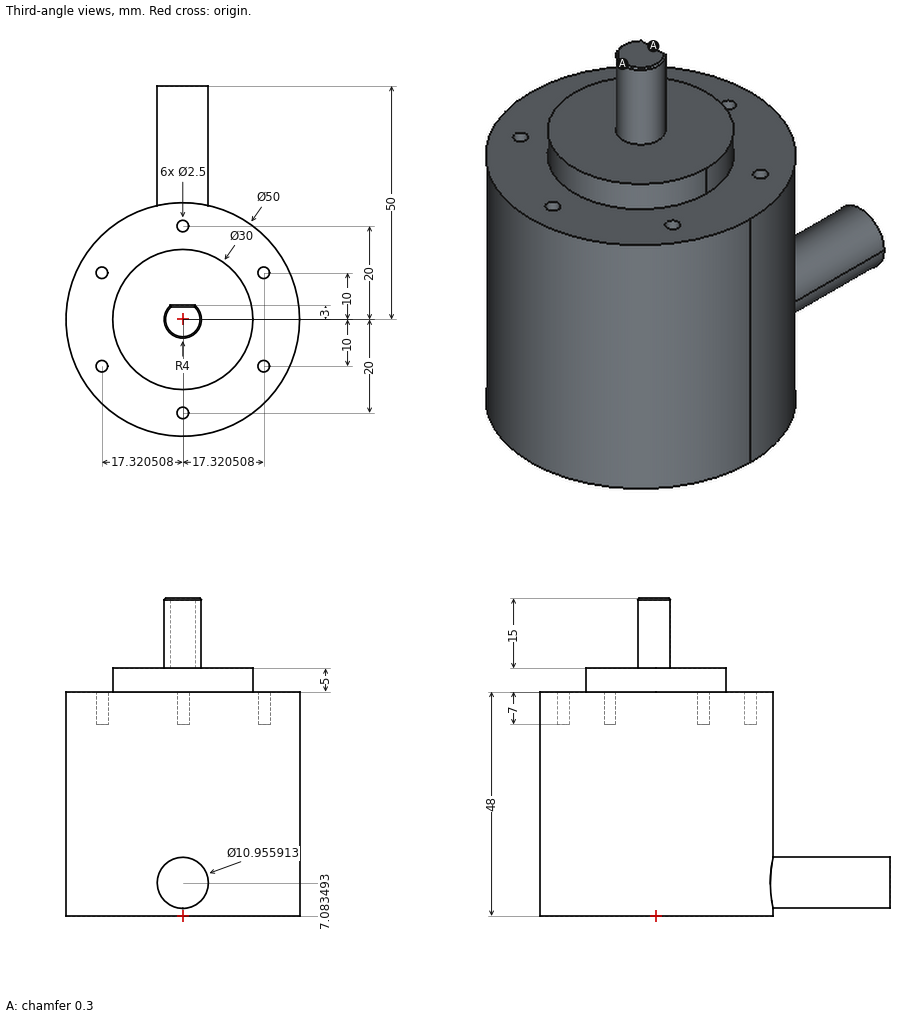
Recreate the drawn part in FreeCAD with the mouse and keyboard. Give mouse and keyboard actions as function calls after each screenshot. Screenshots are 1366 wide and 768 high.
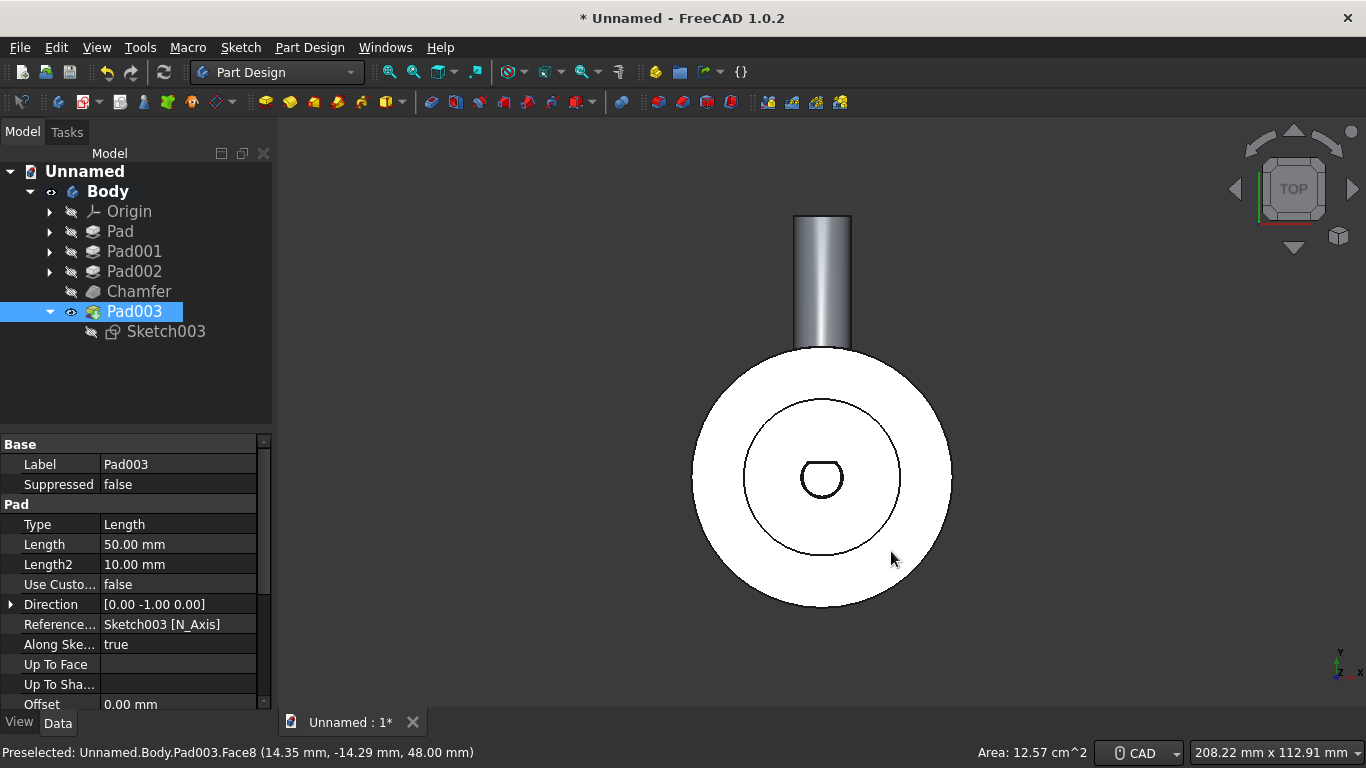
click(84, 102)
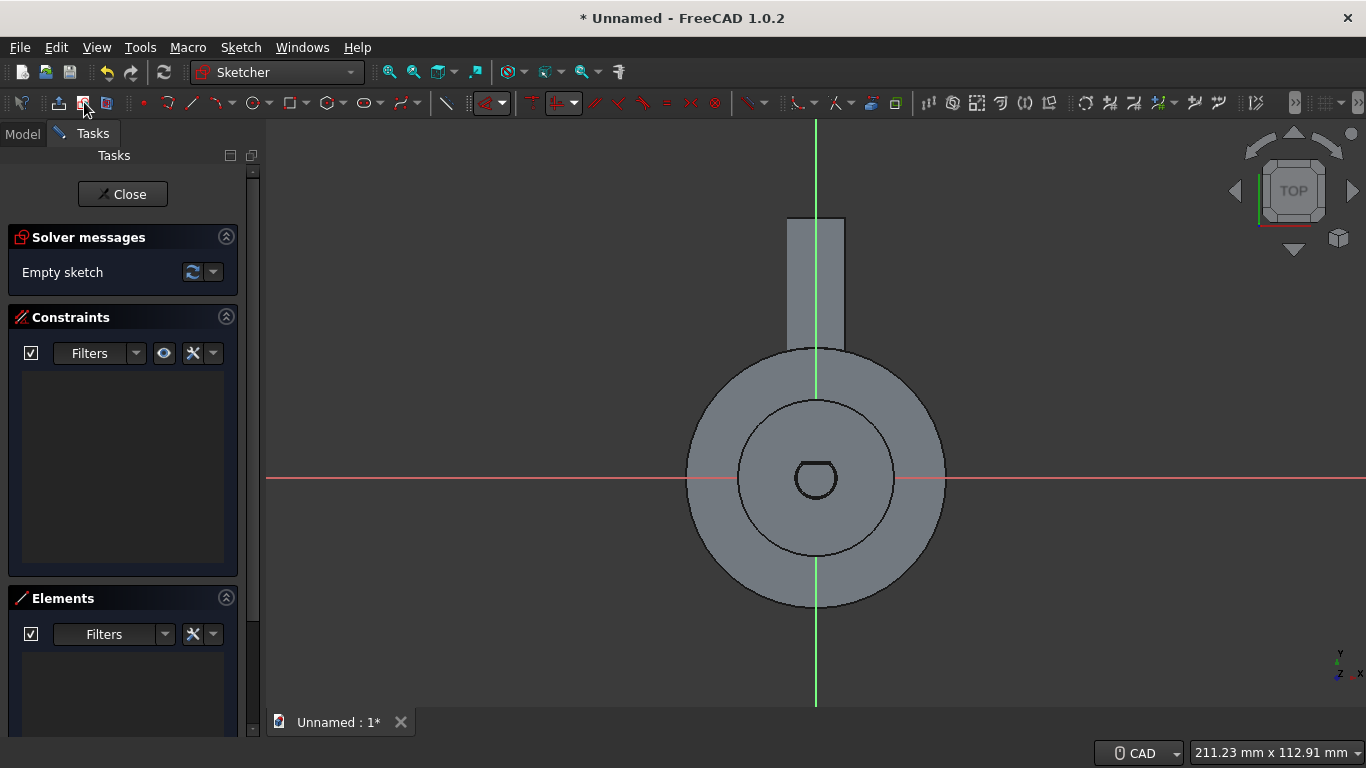
click(108, 104)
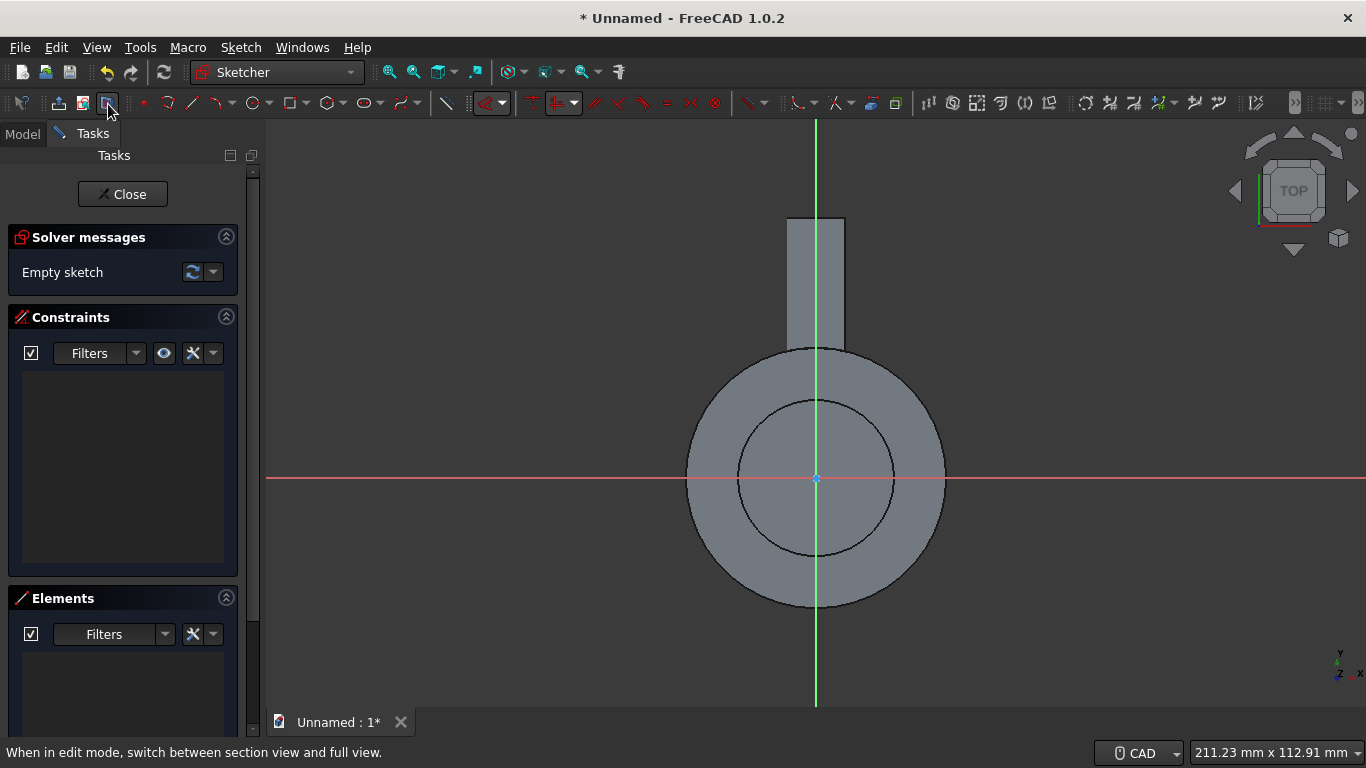
scroll(899, 557, up, 3)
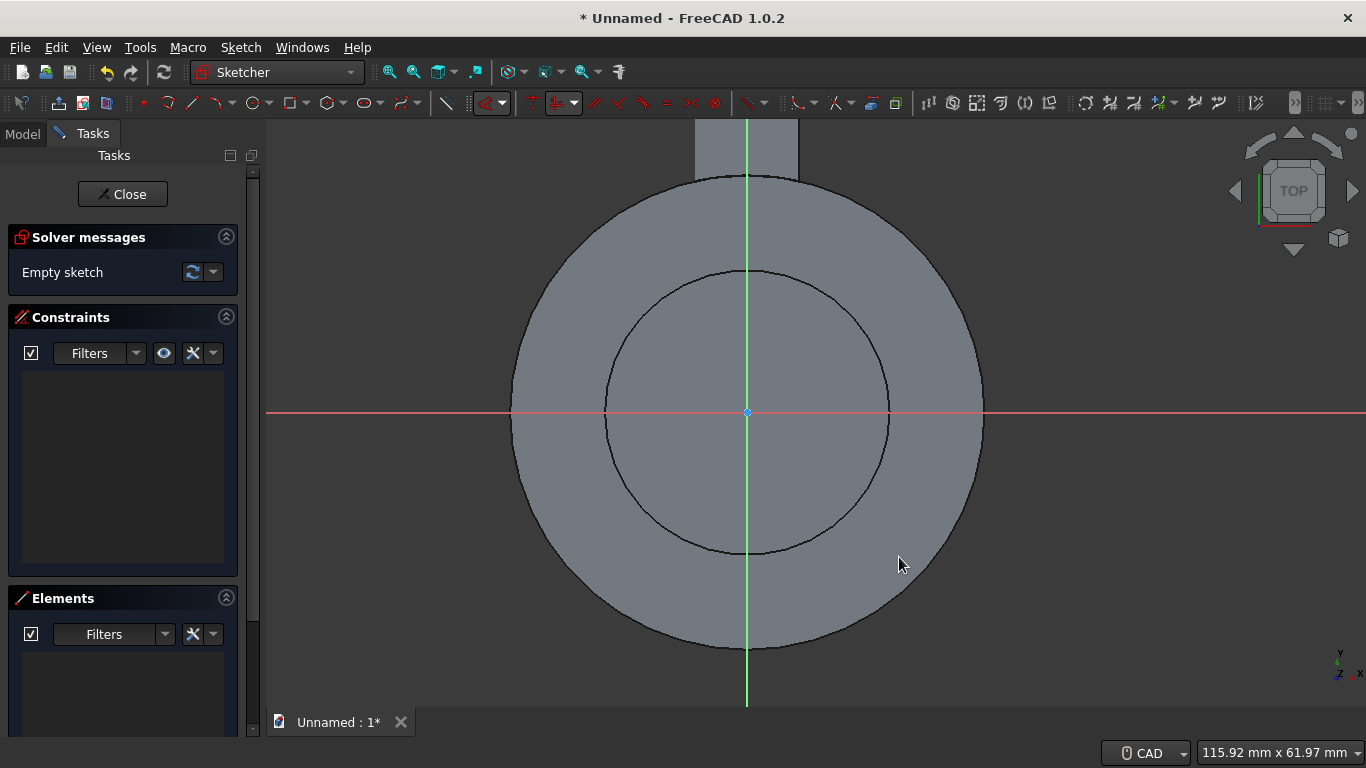
click(254, 104)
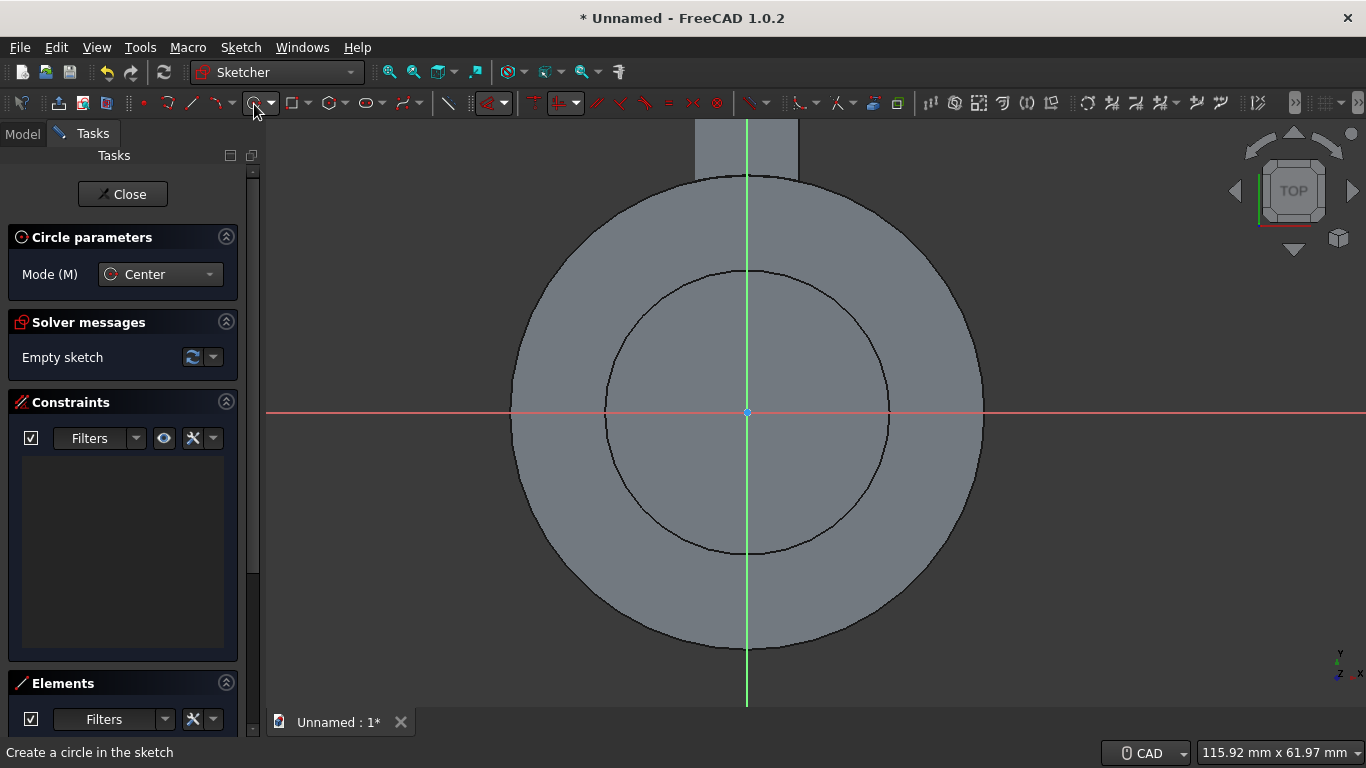
scroll(747, 223, up, 4)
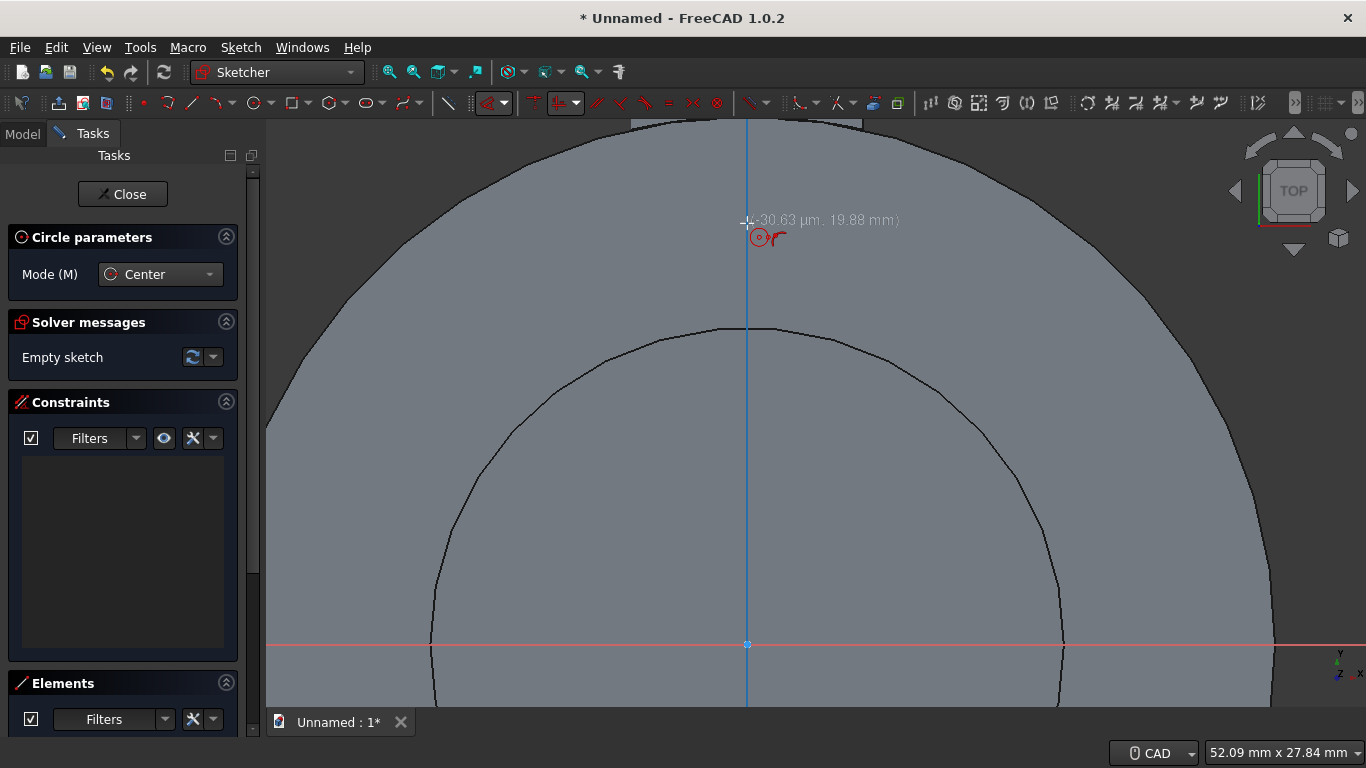
click(747, 222)
move(766, 204)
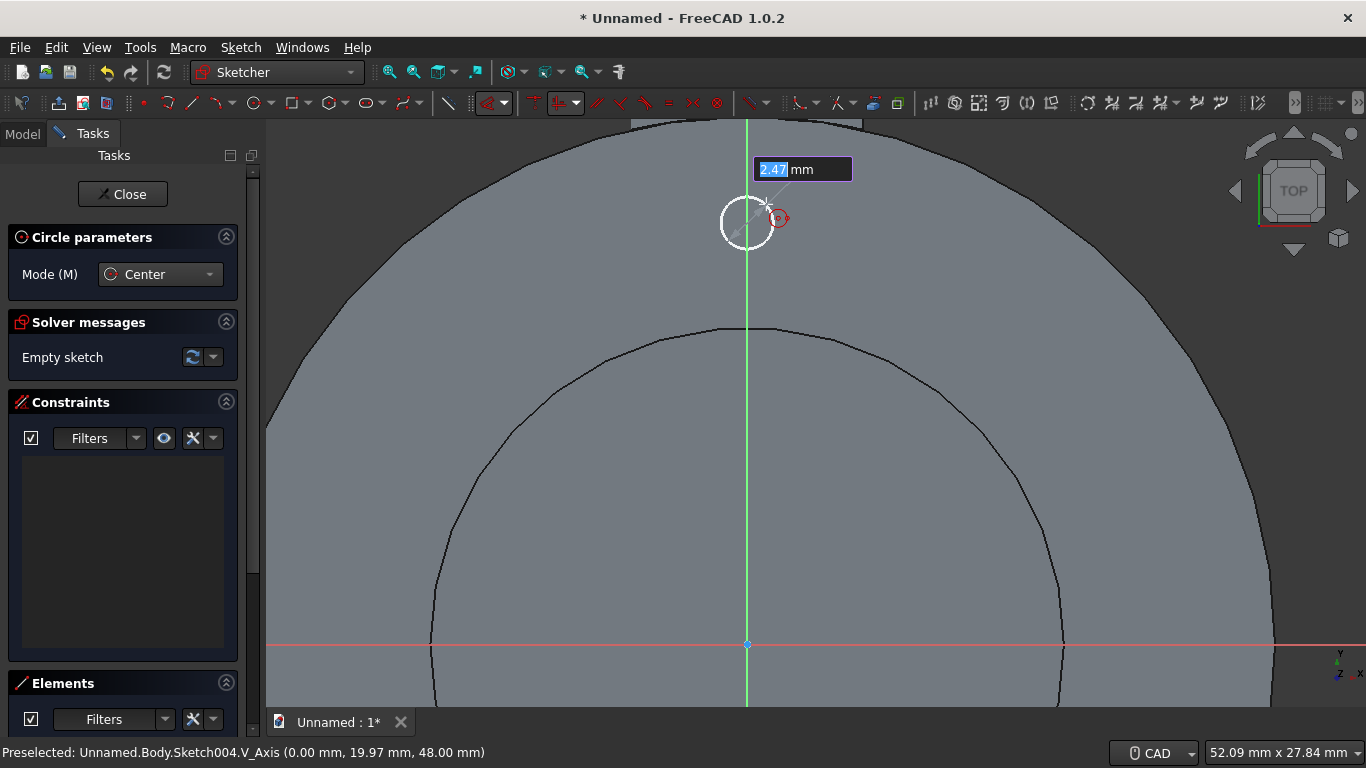
text(2.5)
key(Return)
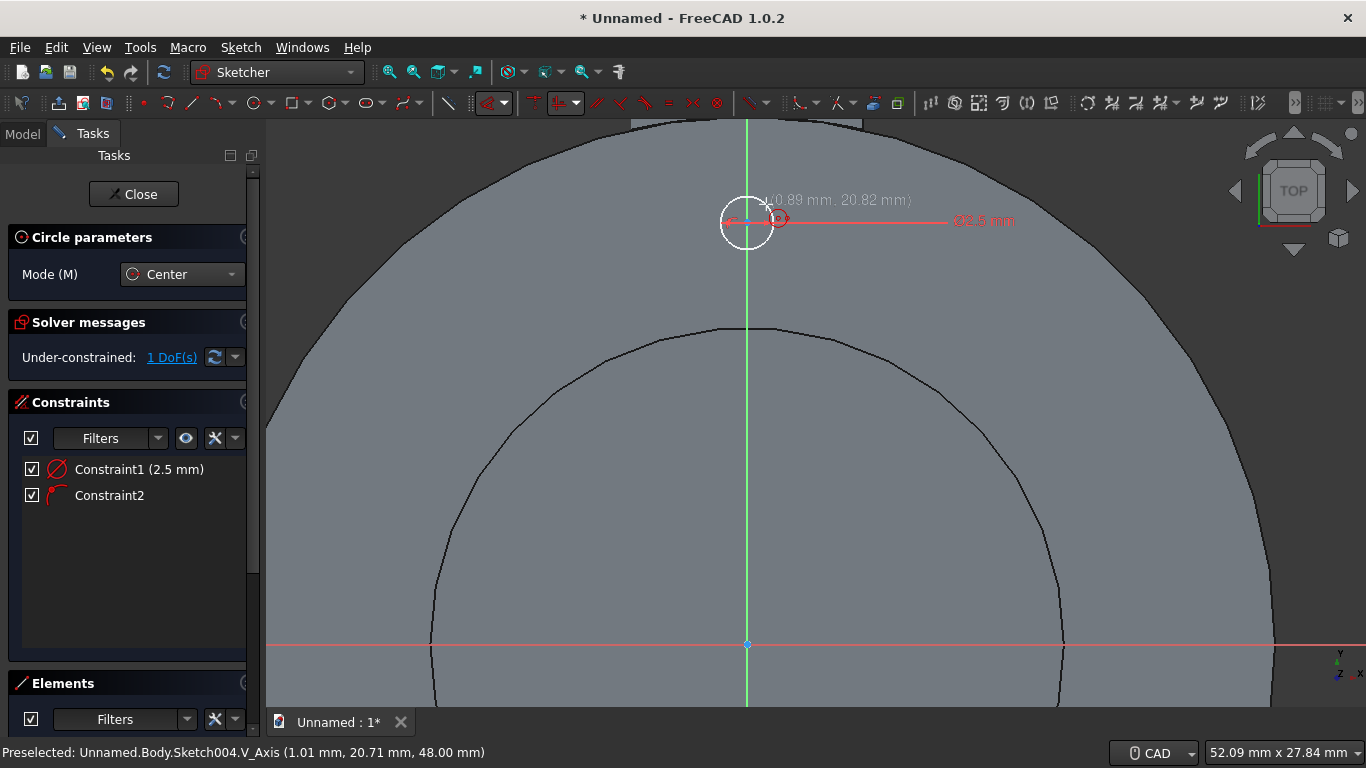
click(1113, 434)
move(1132, 415)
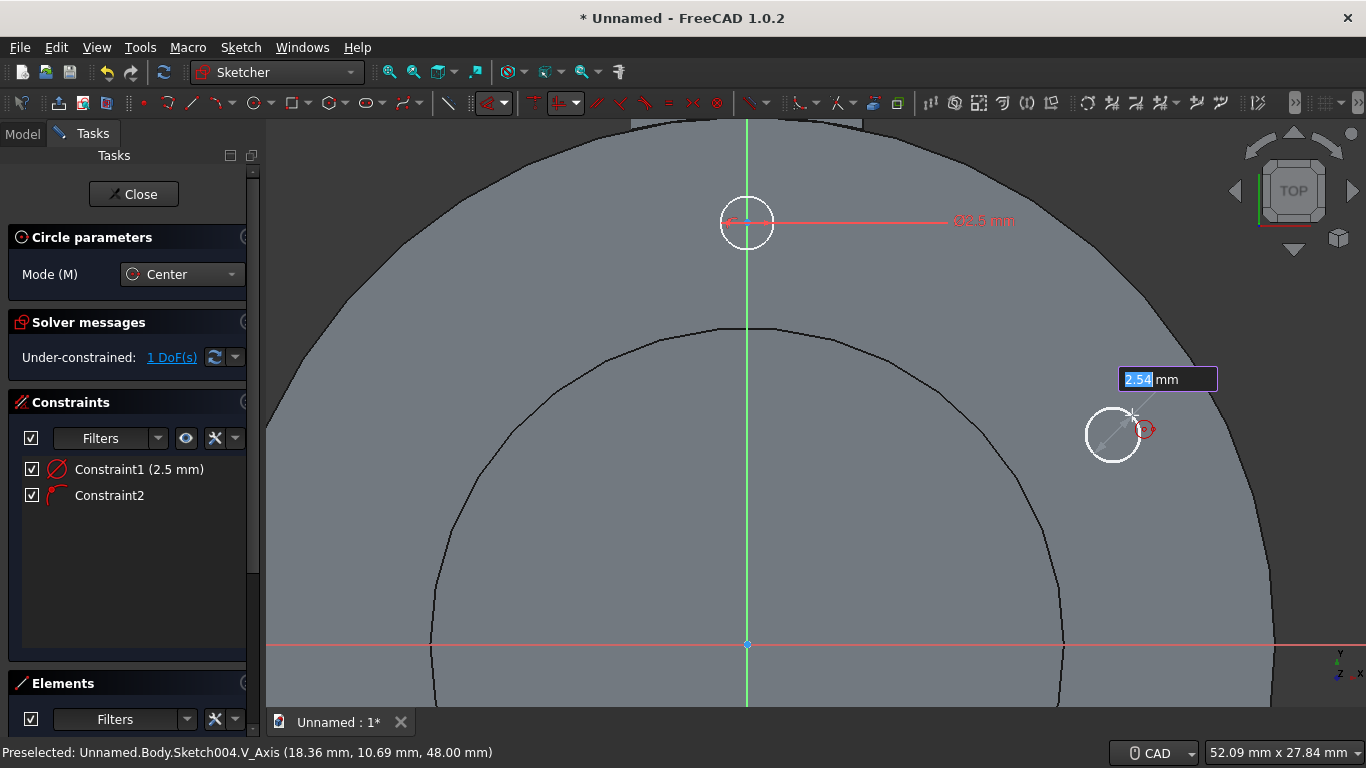
text(2.5)
key(Return)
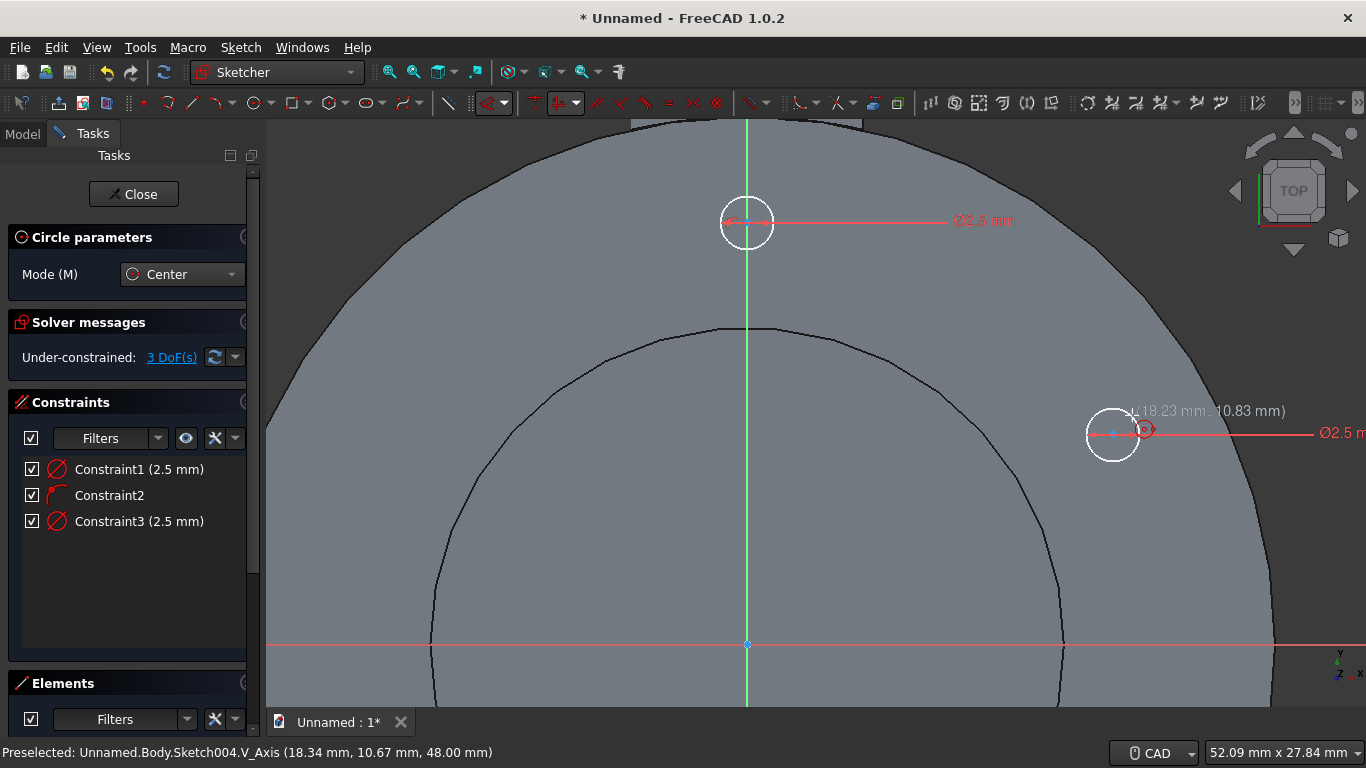
scroll(748, 224, down, 4)